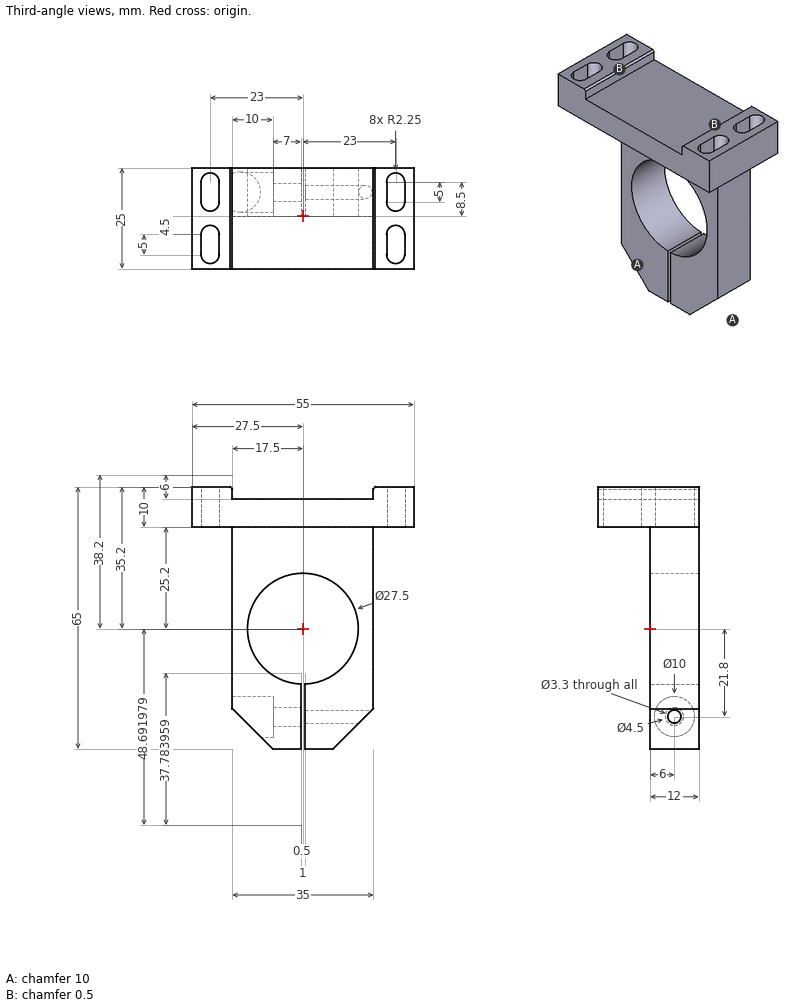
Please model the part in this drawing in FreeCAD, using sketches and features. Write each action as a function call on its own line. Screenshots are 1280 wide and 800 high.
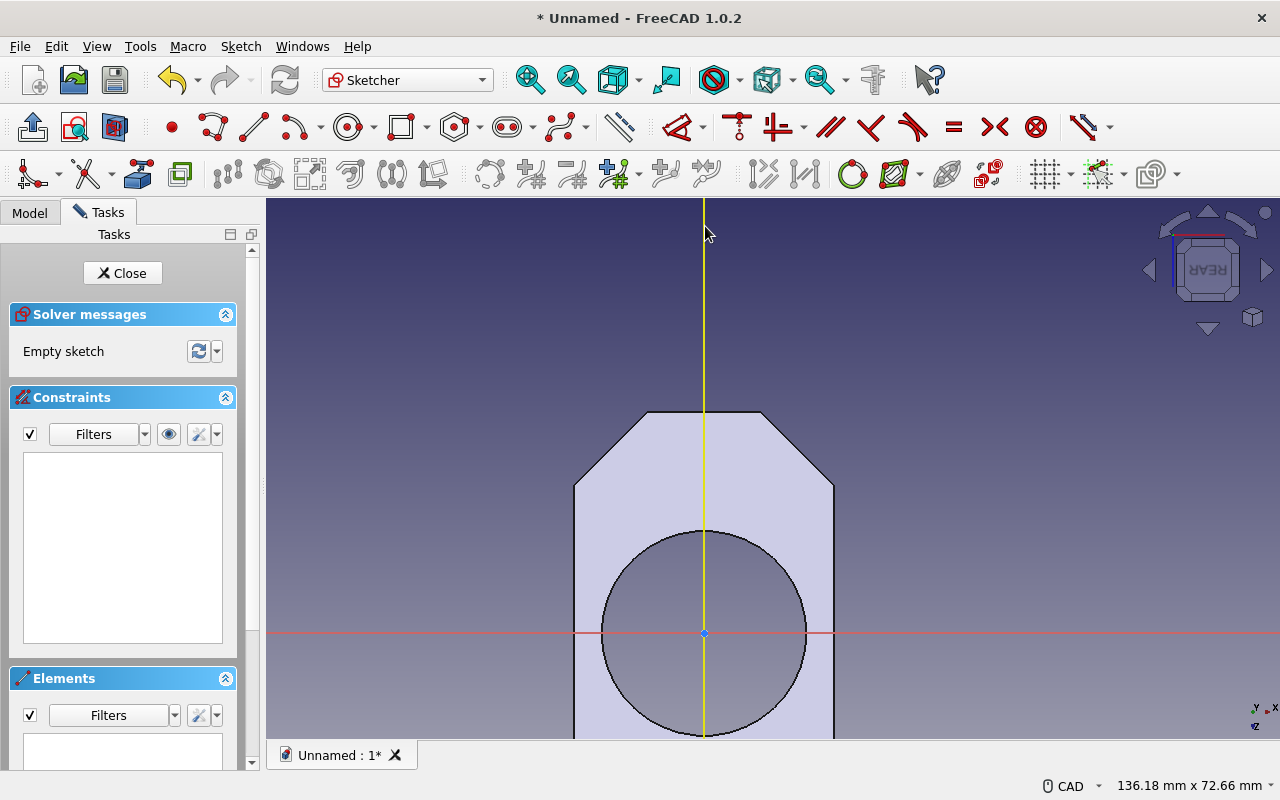
key(g)
key(r)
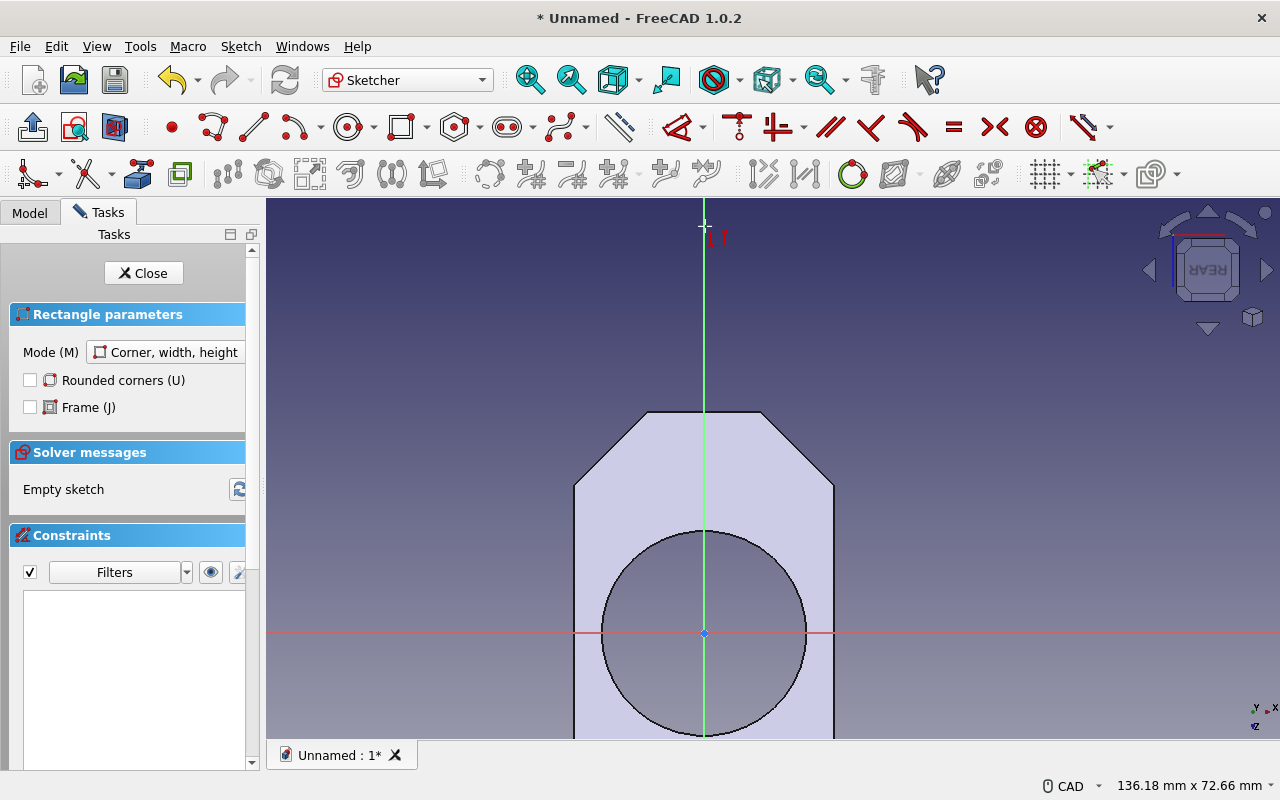
scroll(700, 271, up, 8)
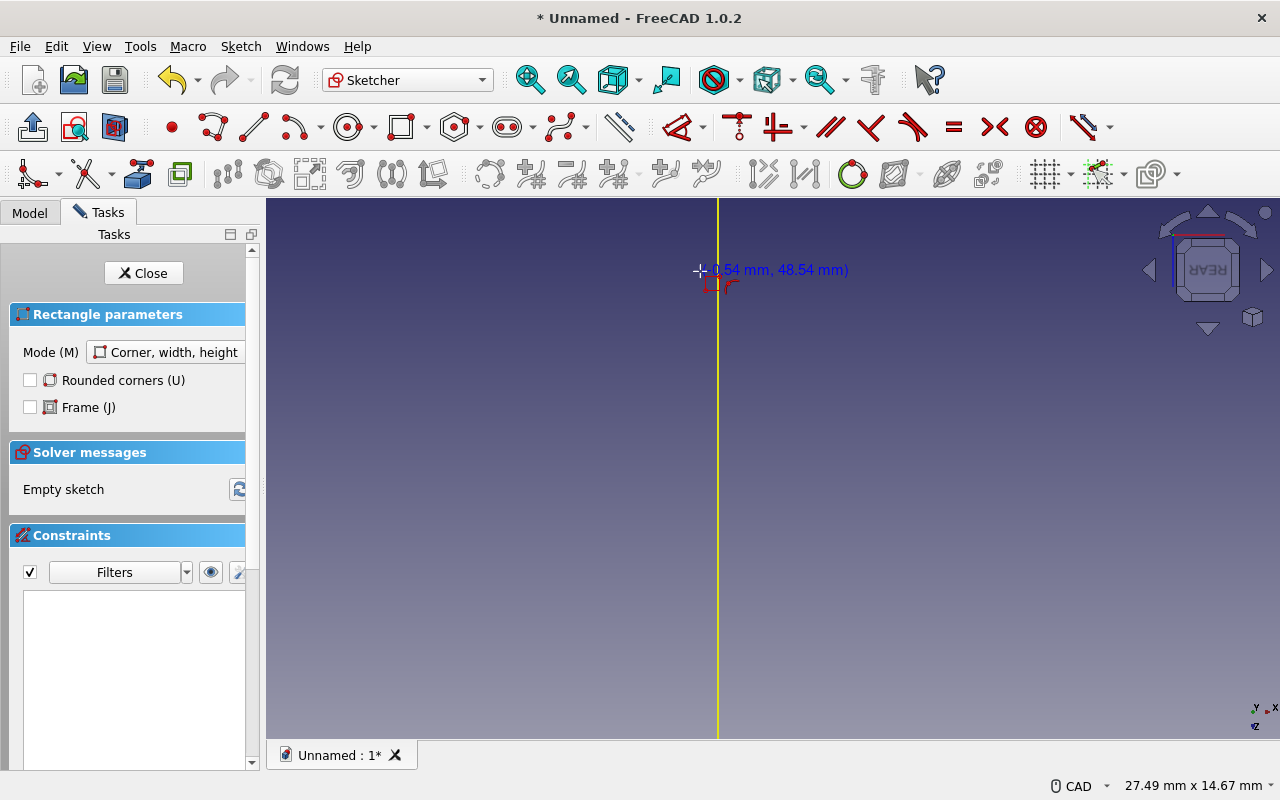
click(700, 270)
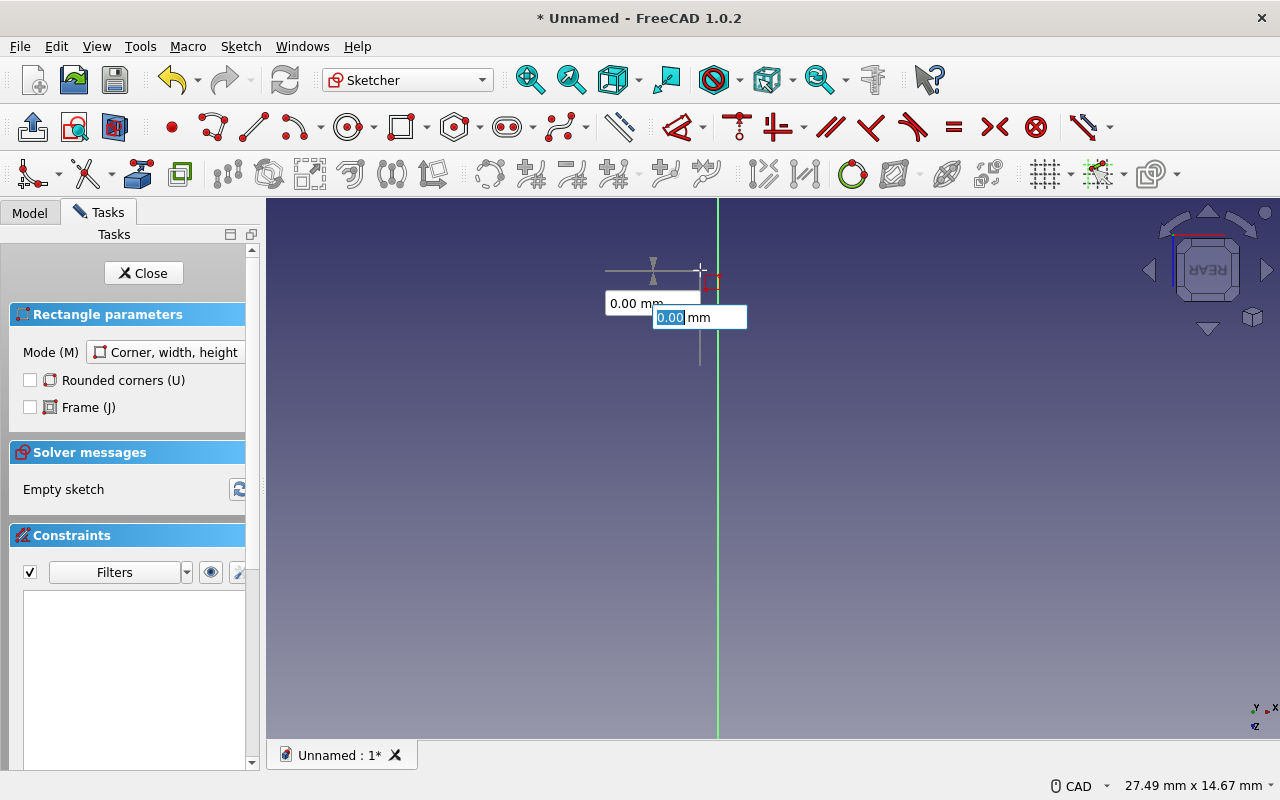
scroll(701, 292, down, 8)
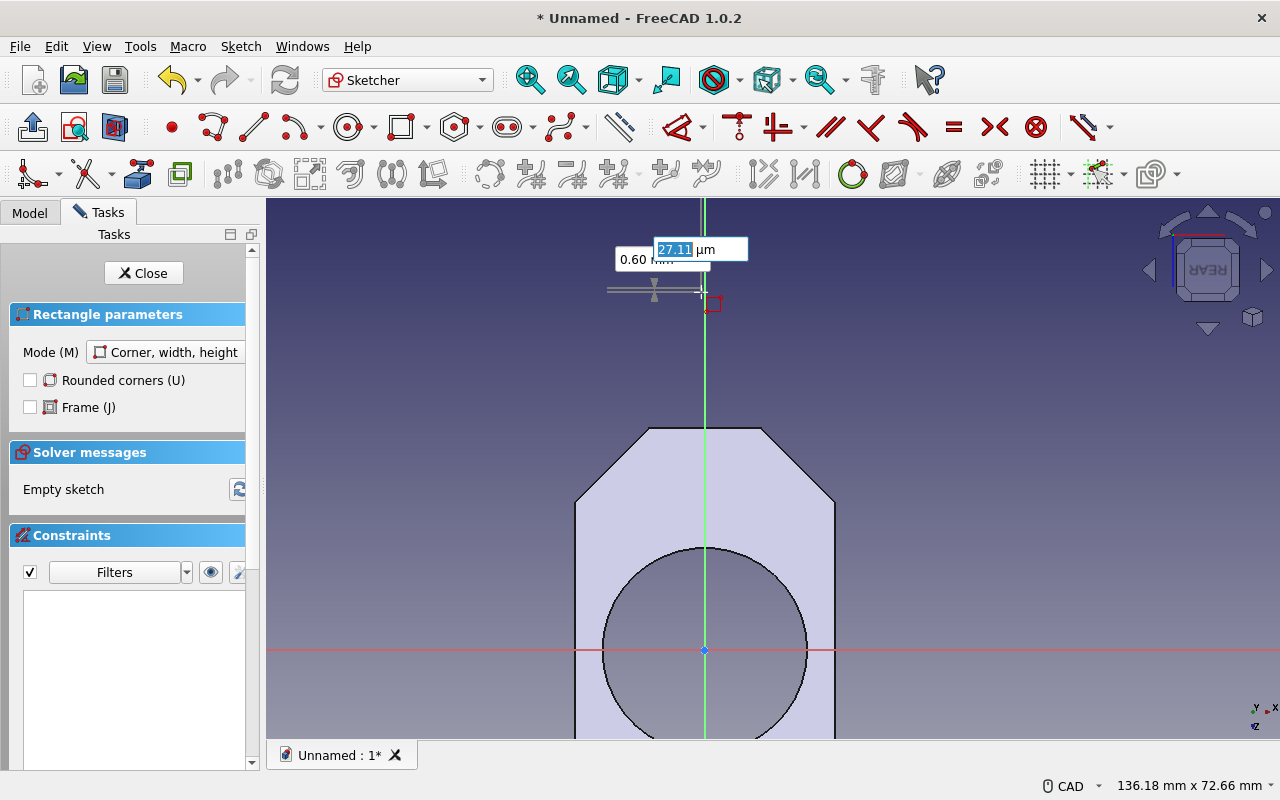
scroll(709, 569, up, 8)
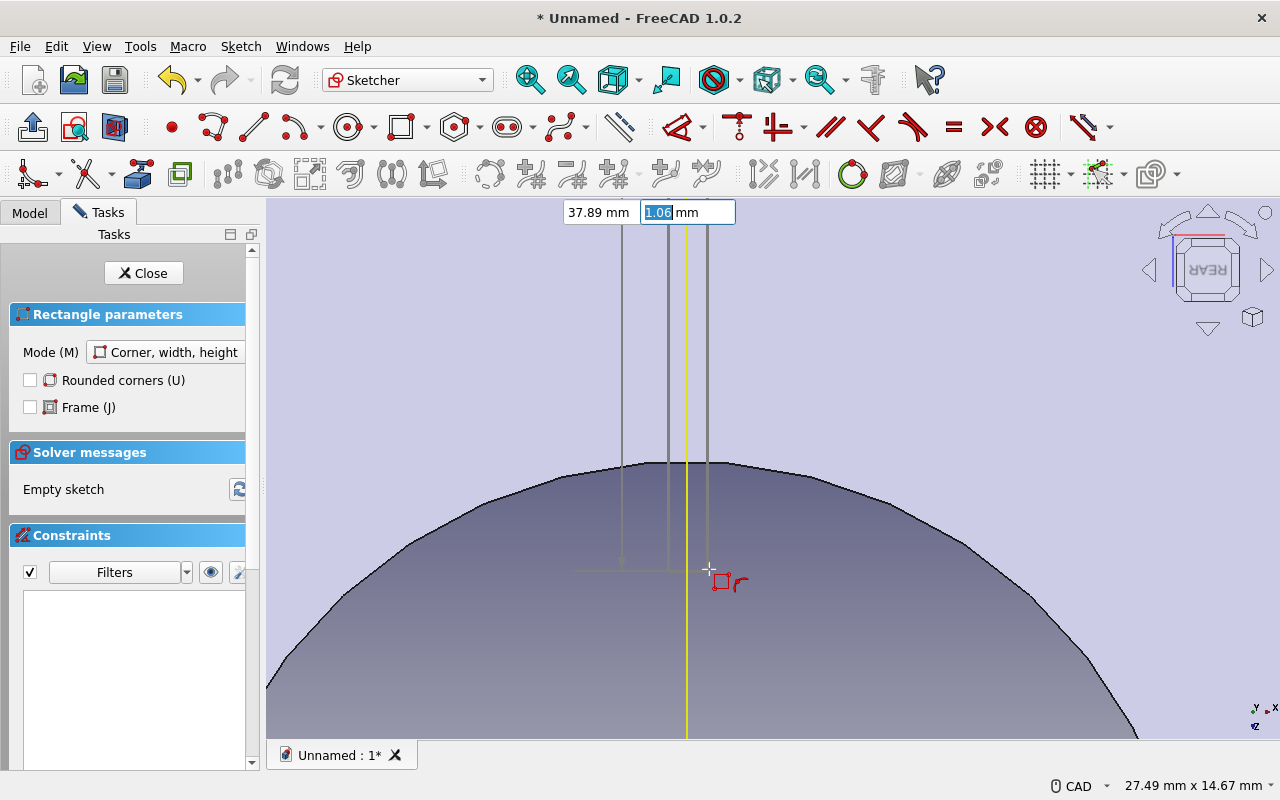
click(705, 566)
key(Escape)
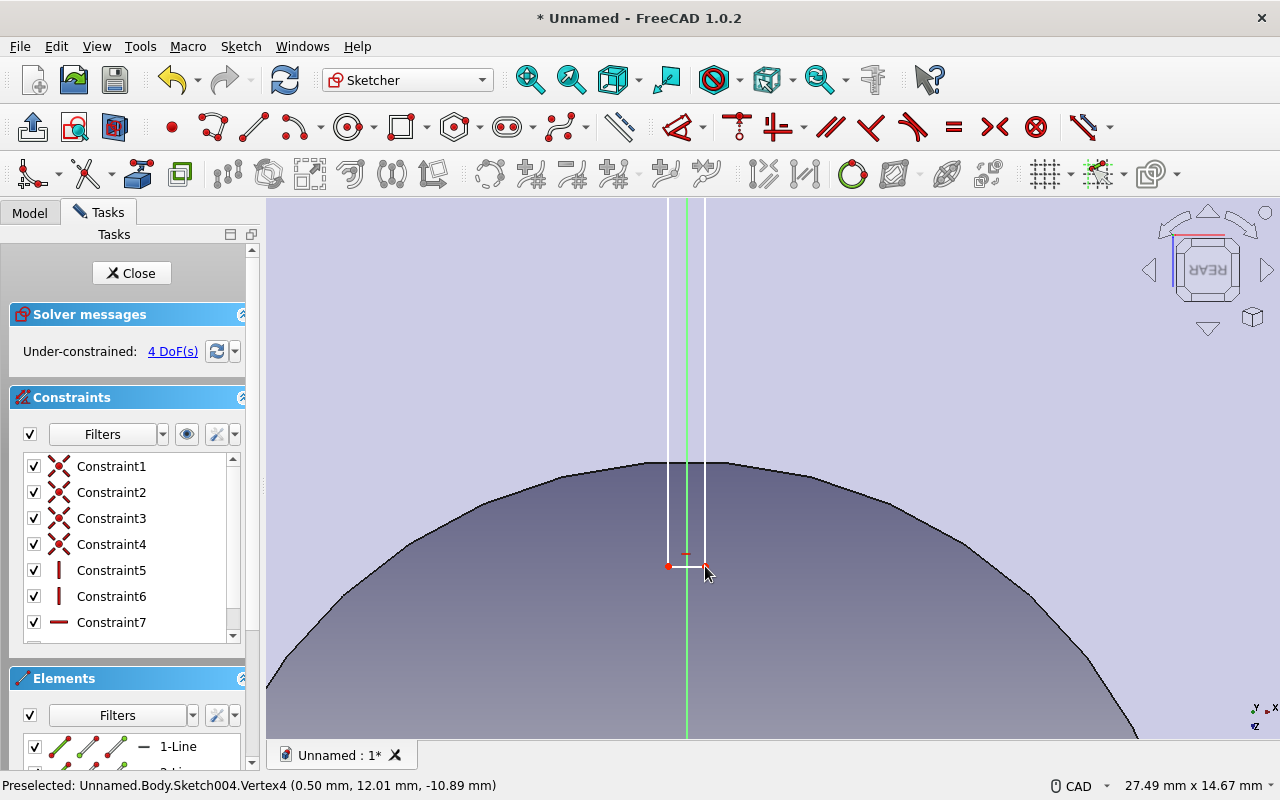
click(676, 128)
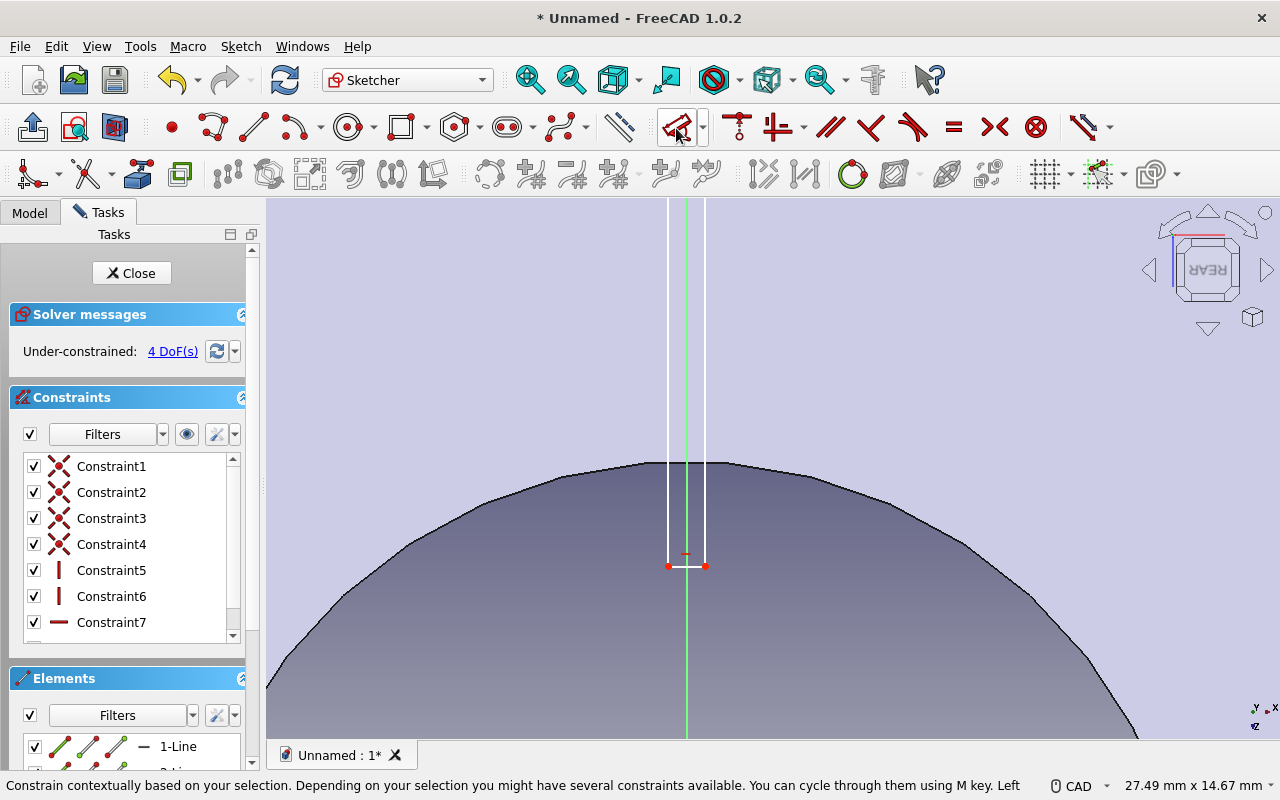
click(683, 567)
click(678, 601)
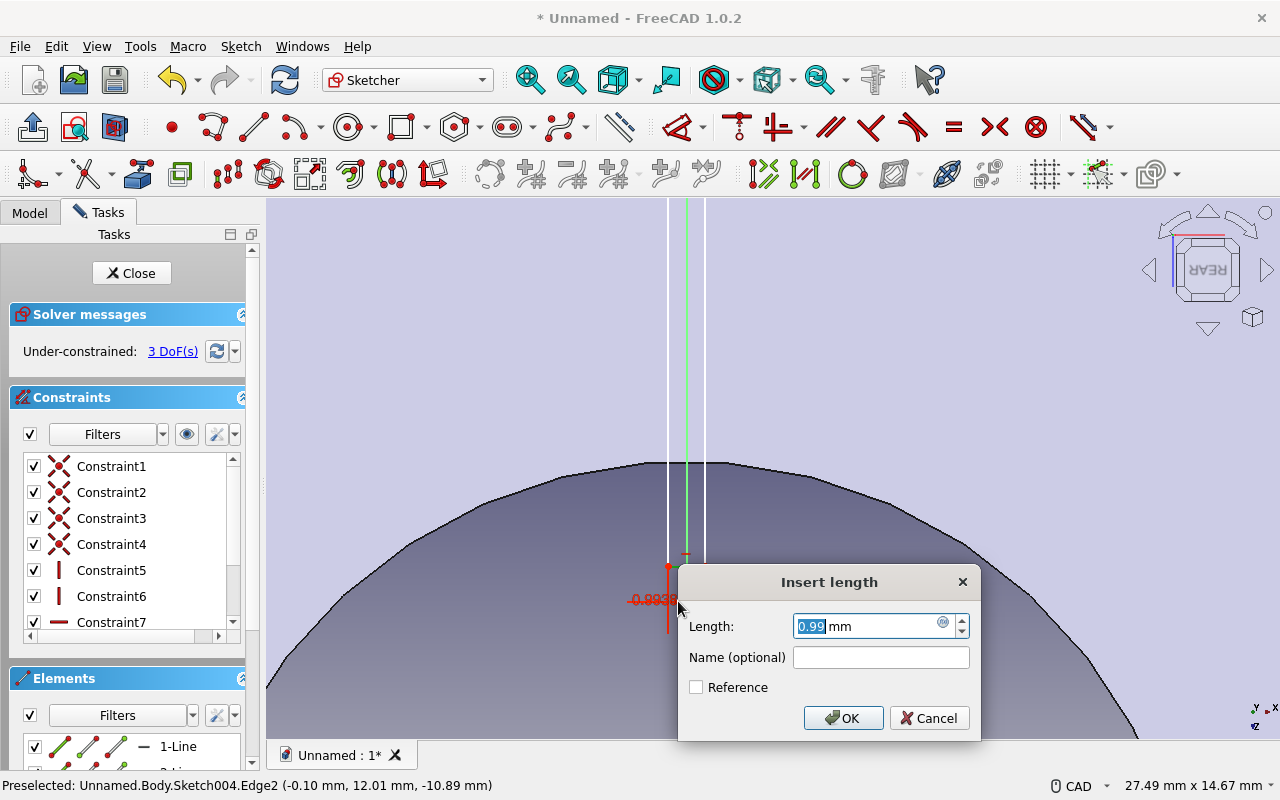
text(1)
key(Return)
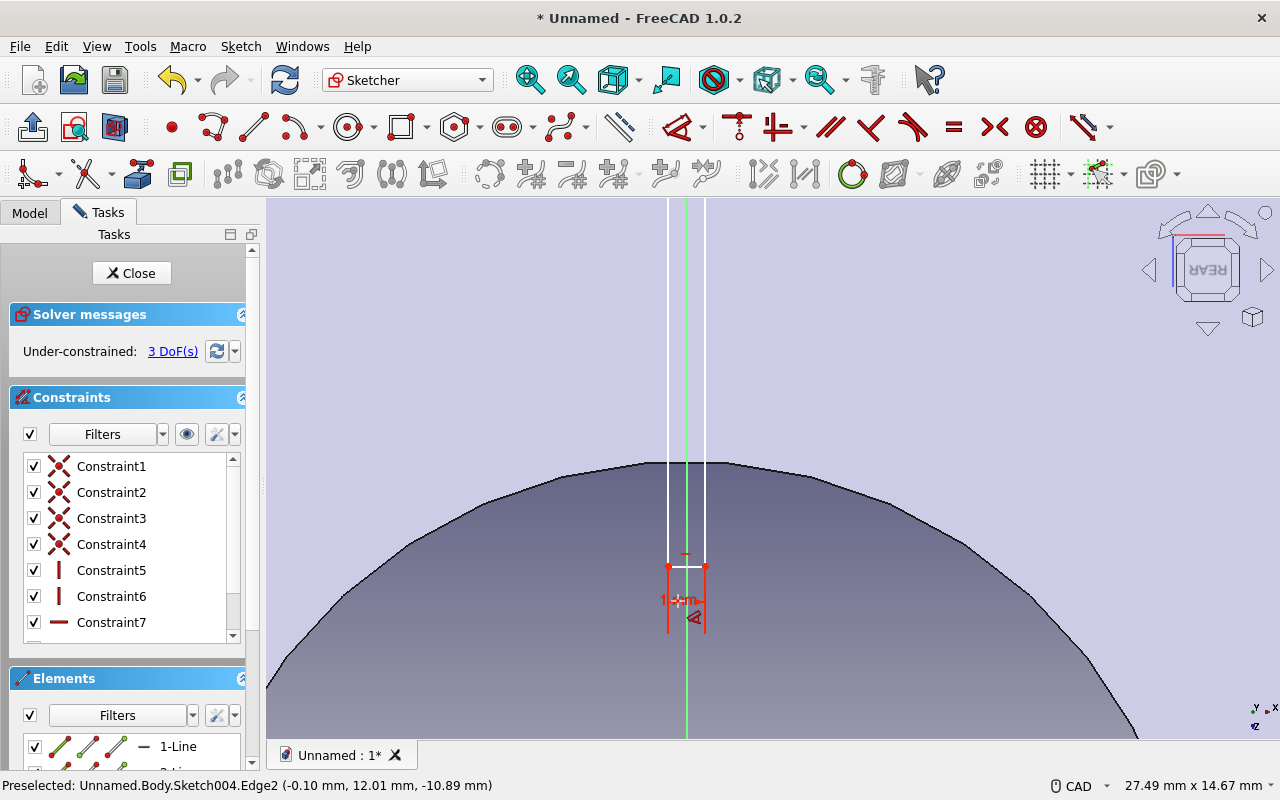
scroll(709, 569, down, 8)